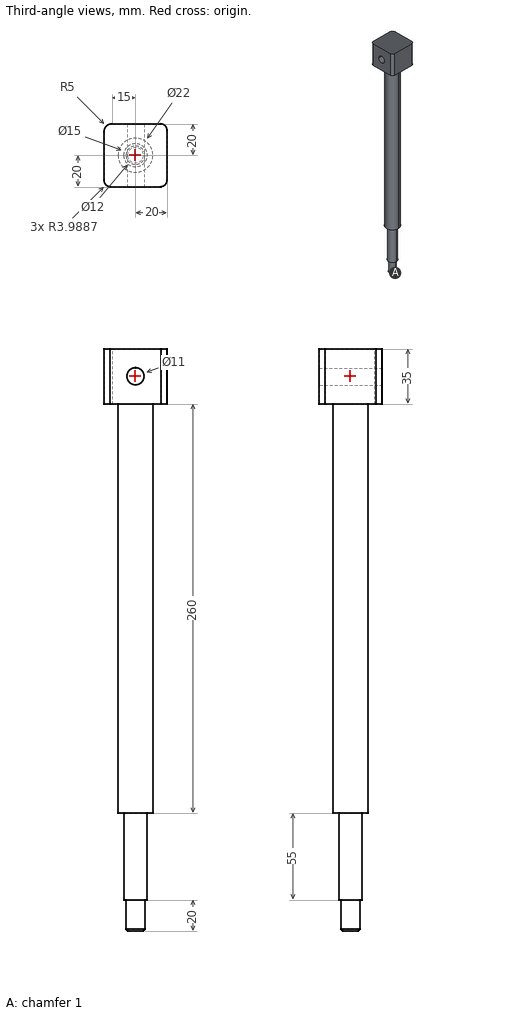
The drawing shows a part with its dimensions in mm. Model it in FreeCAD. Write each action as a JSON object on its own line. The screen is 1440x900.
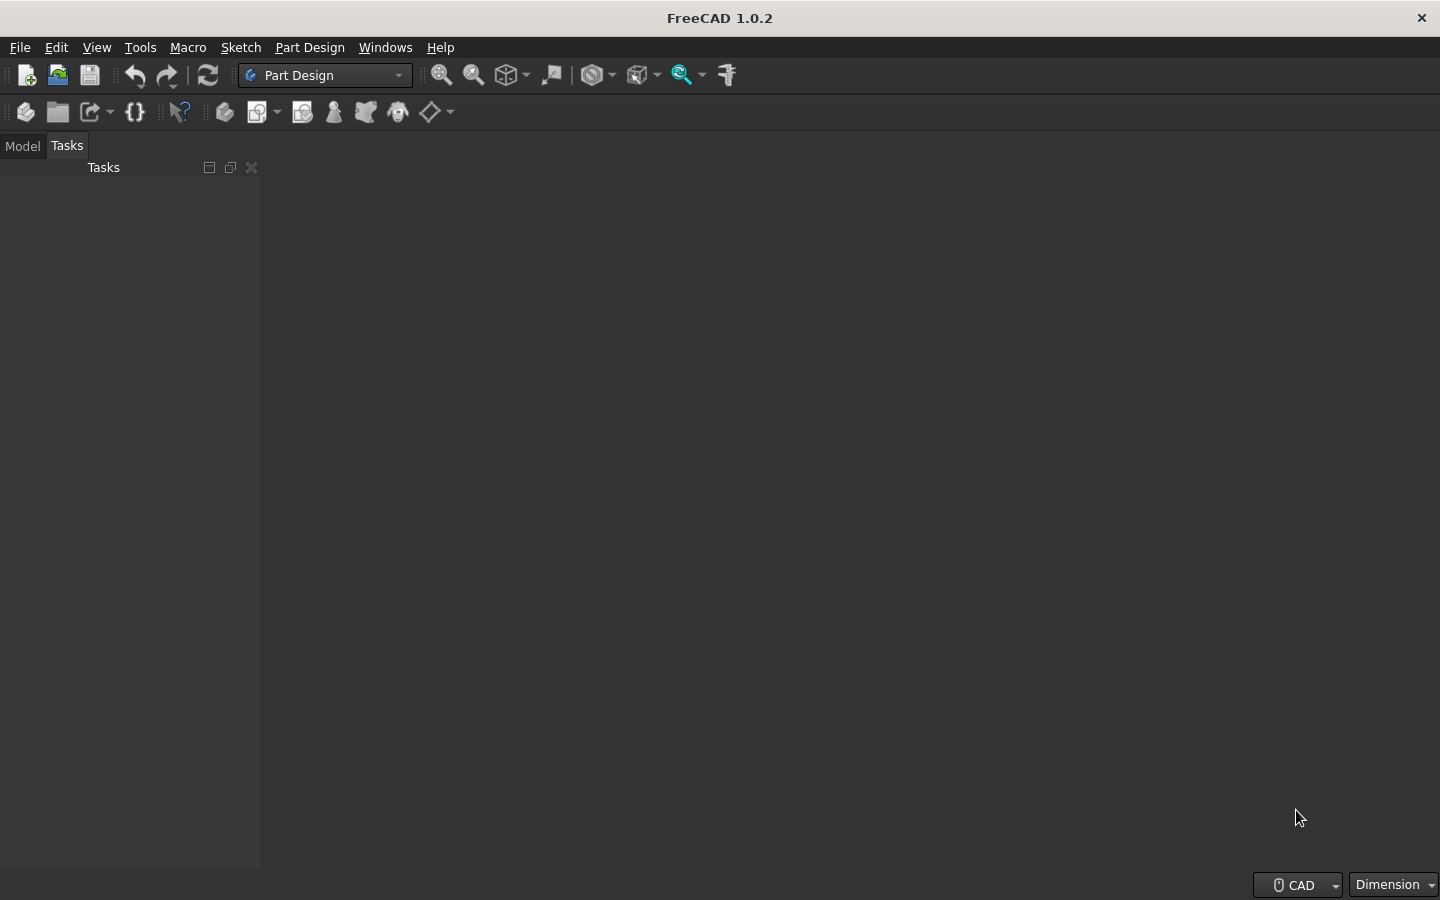
{"action": "left_click", "coordinate": [26, 76]}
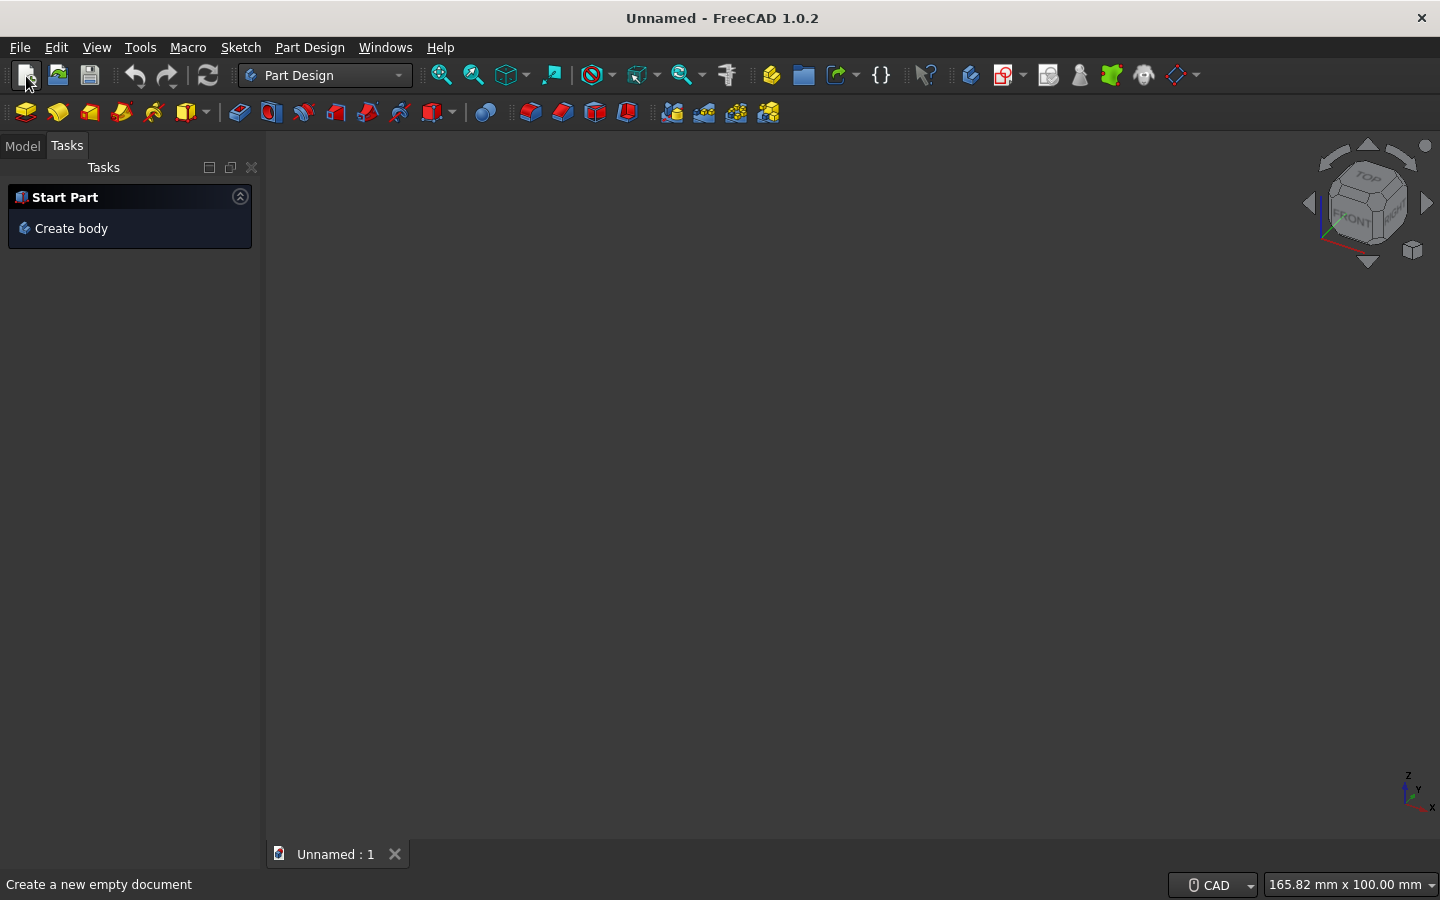
{"action": "left_click", "coordinate": [1004, 76]}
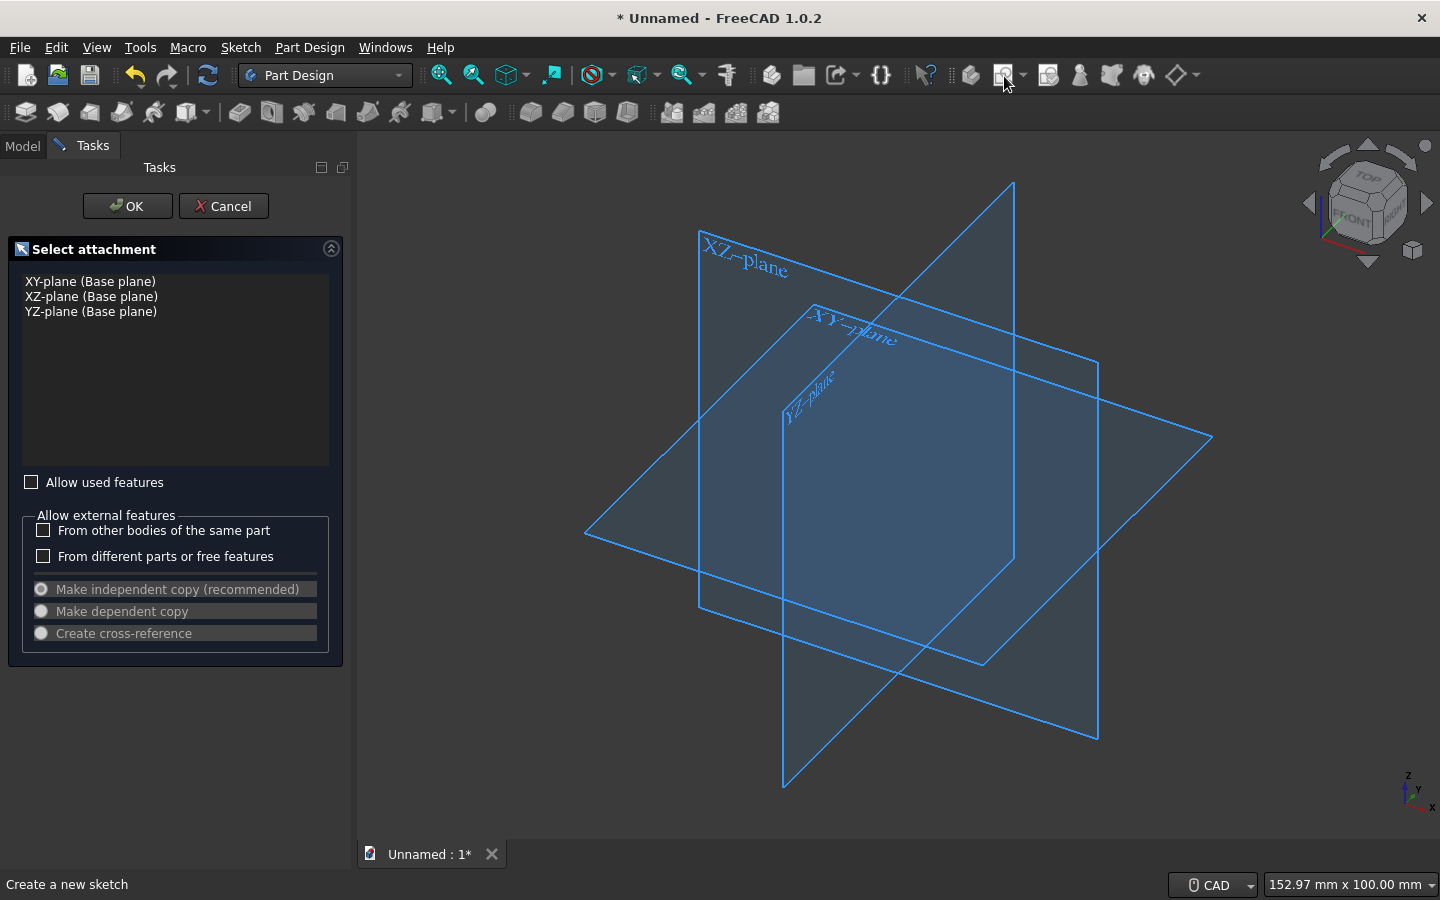
{"action": "left_click", "coordinate": [82, 282]}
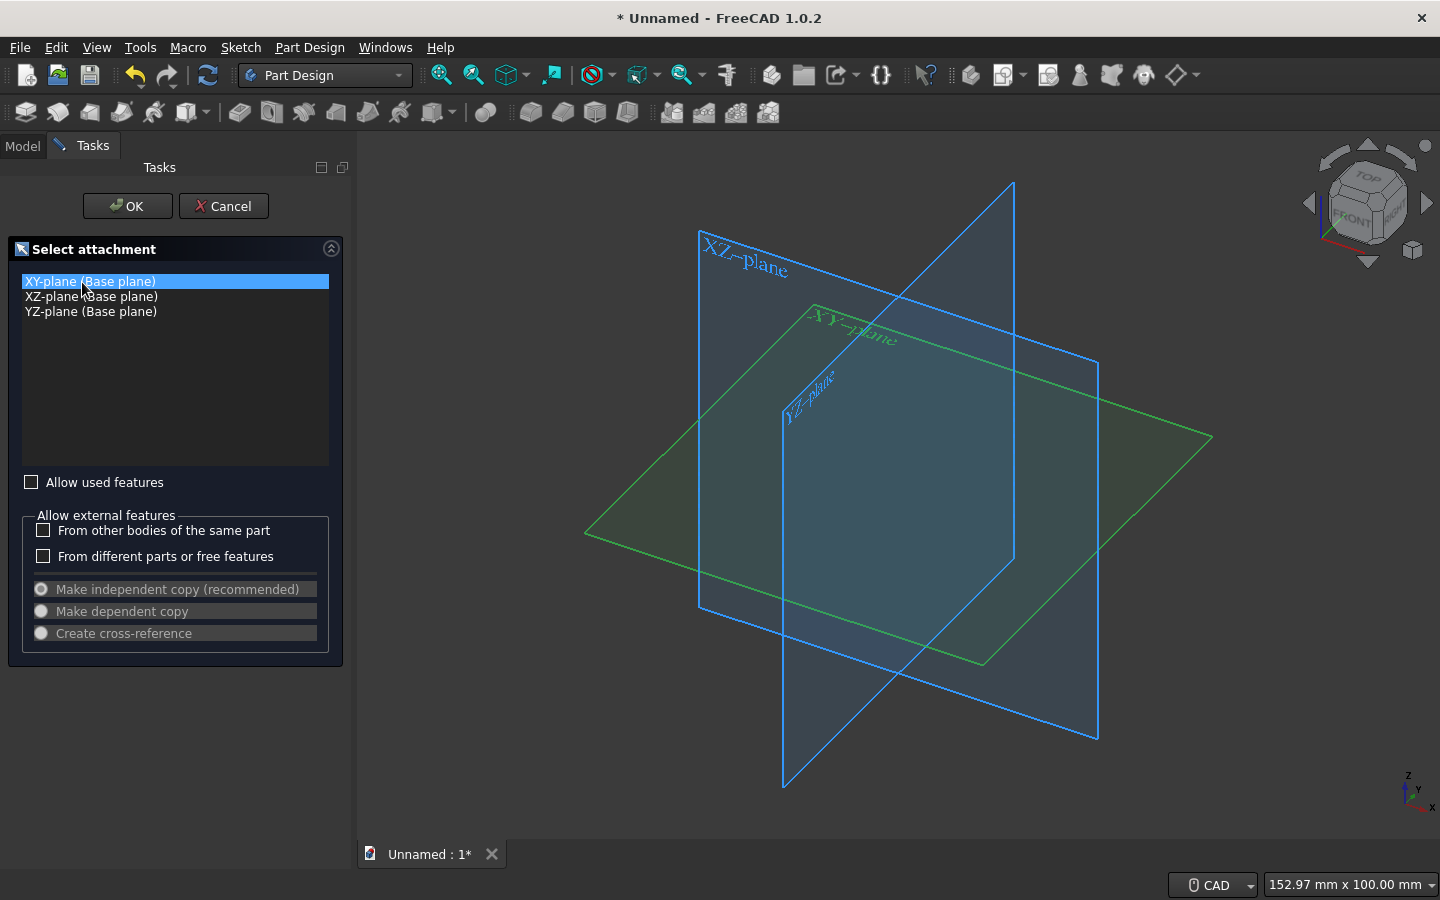
{"action": "left_click", "coordinate": [128, 206]}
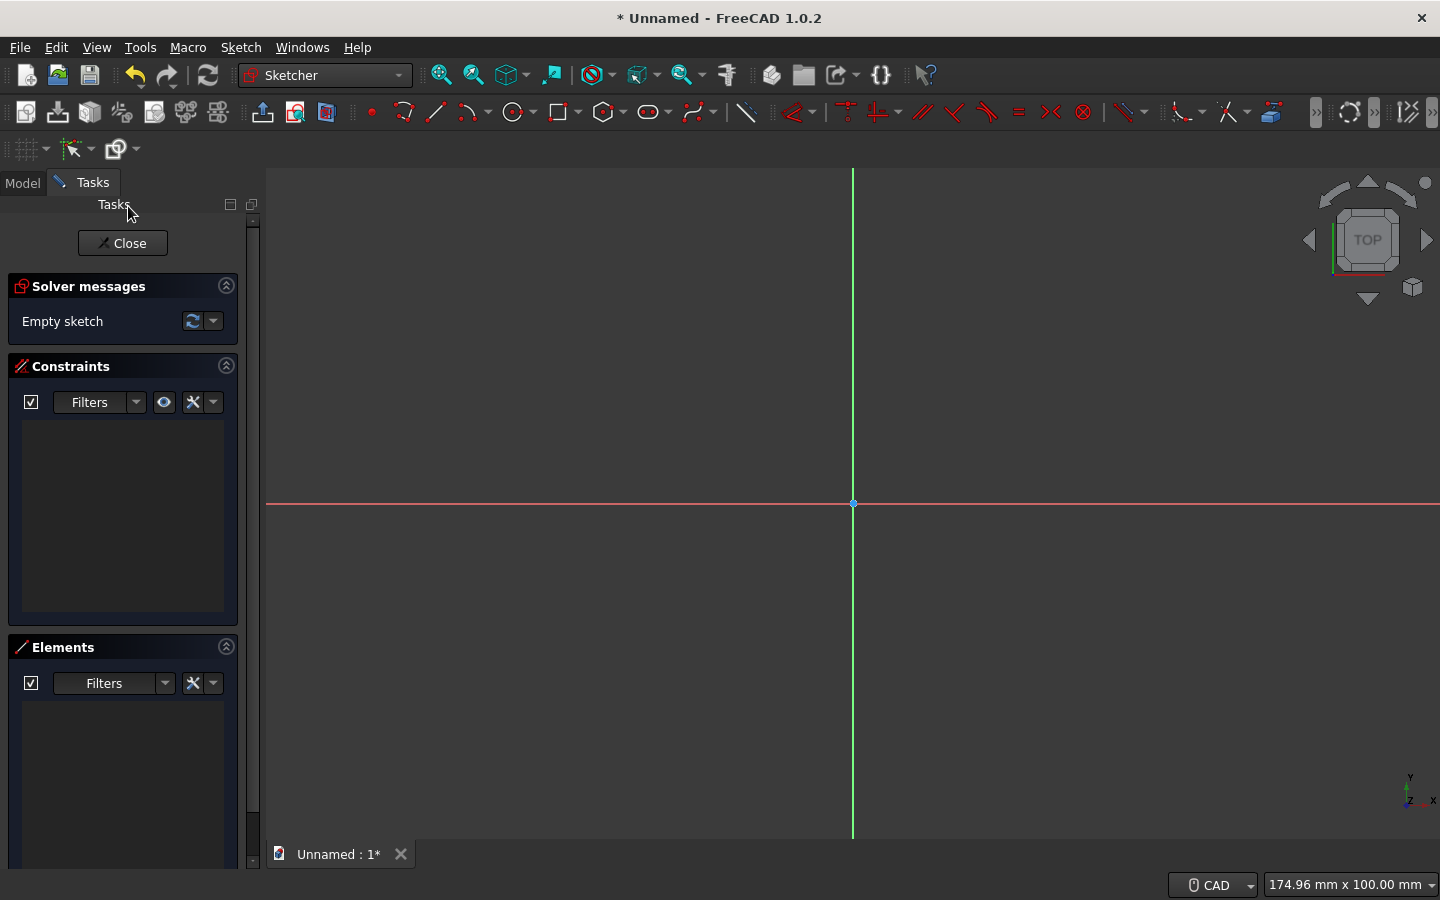
{"action": "scroll", "coordinate": [992, 504], "scroll_direction": "up", "scroll_amount": 2}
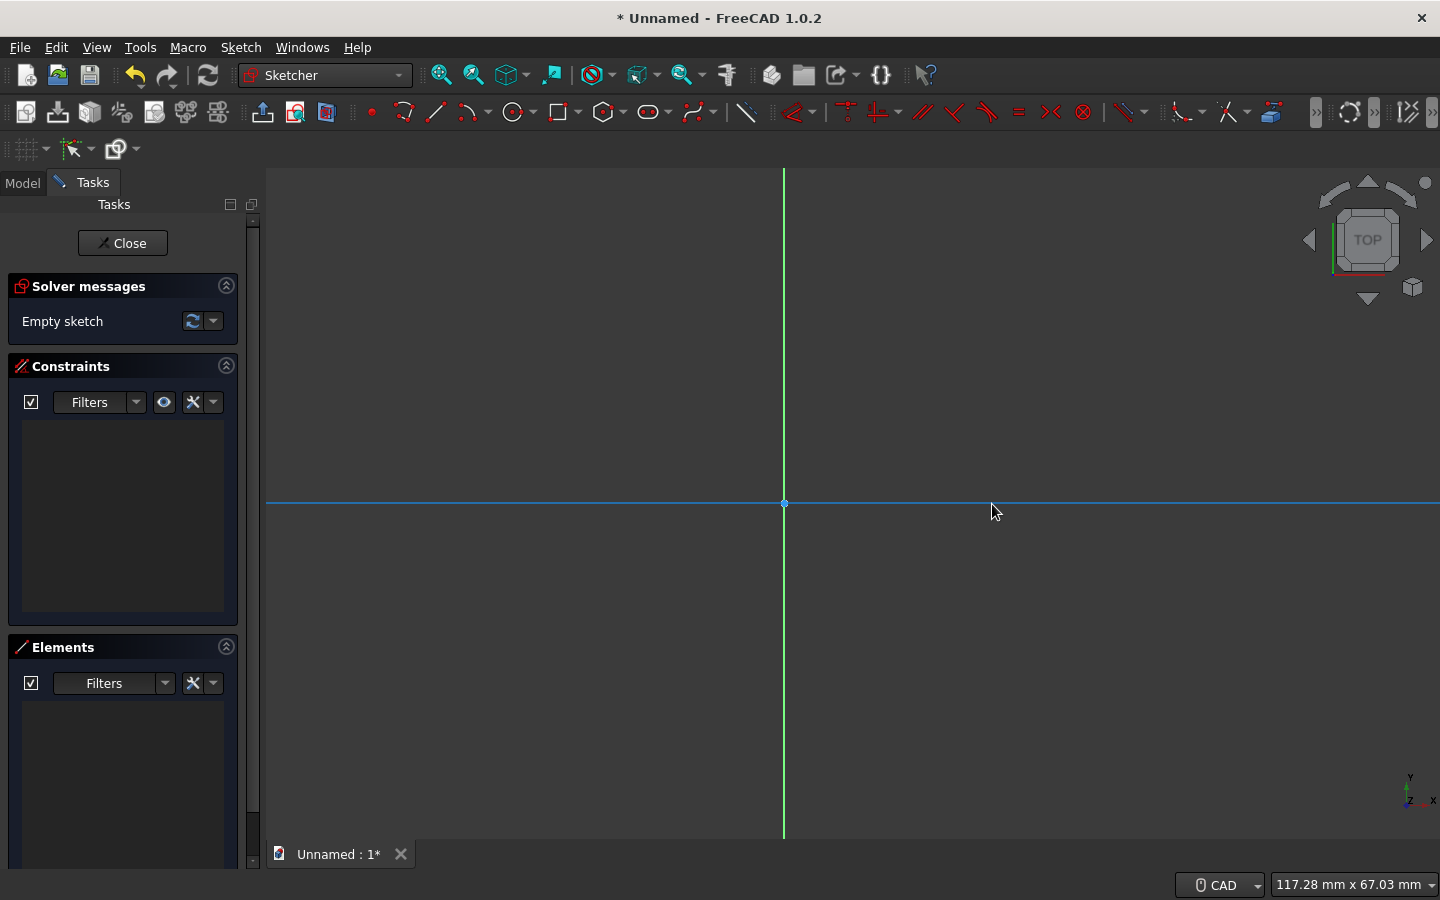
{"action": "key", "text": "g l"}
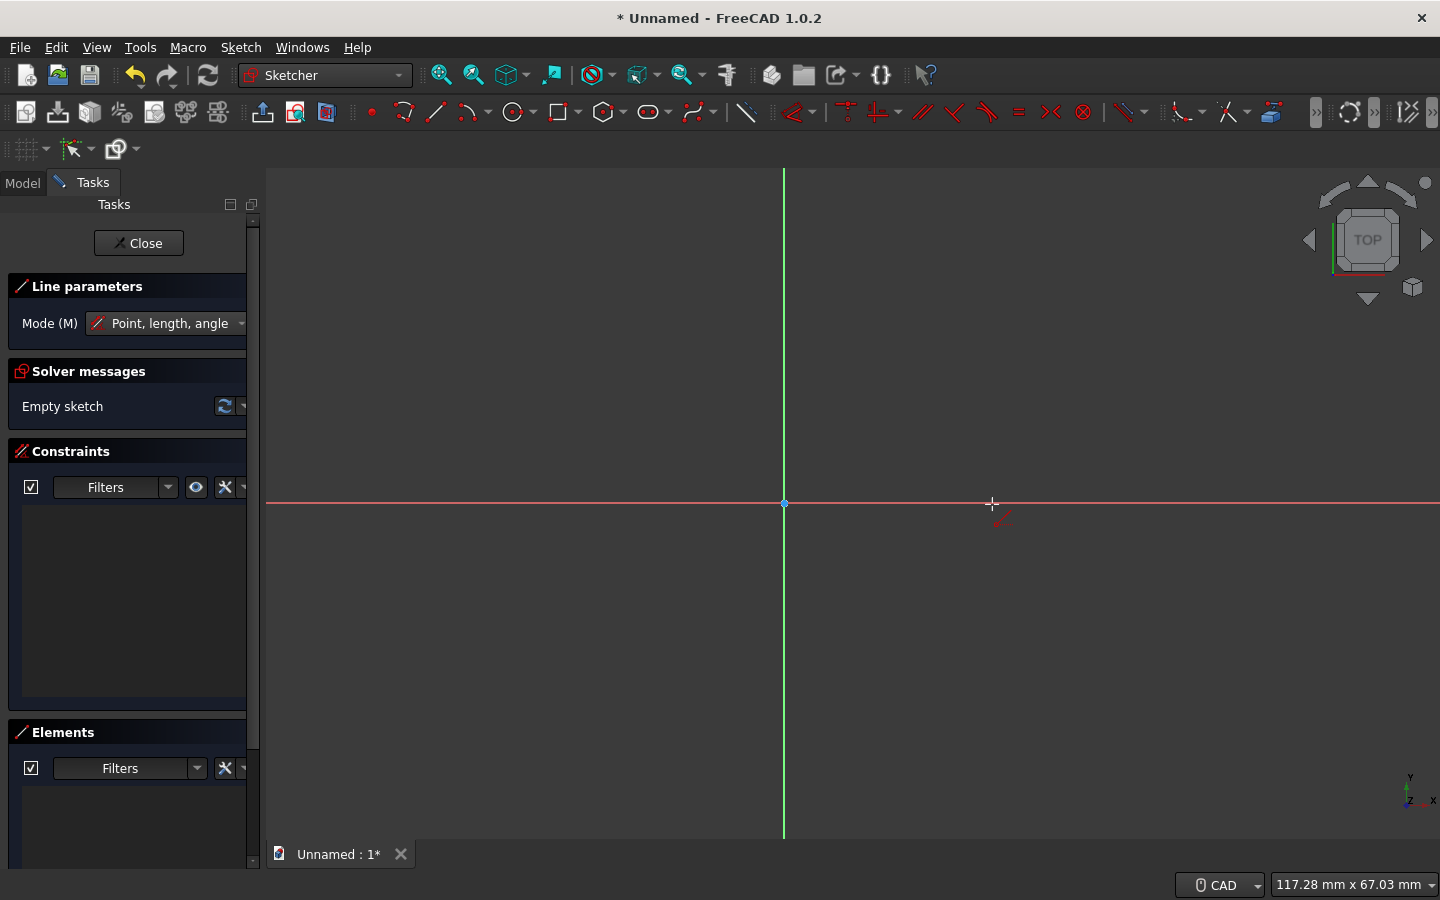
{"action": "left_click", "coordinate": [945, 303]}
{"action": "left_click", "coordinate": [634, 303]}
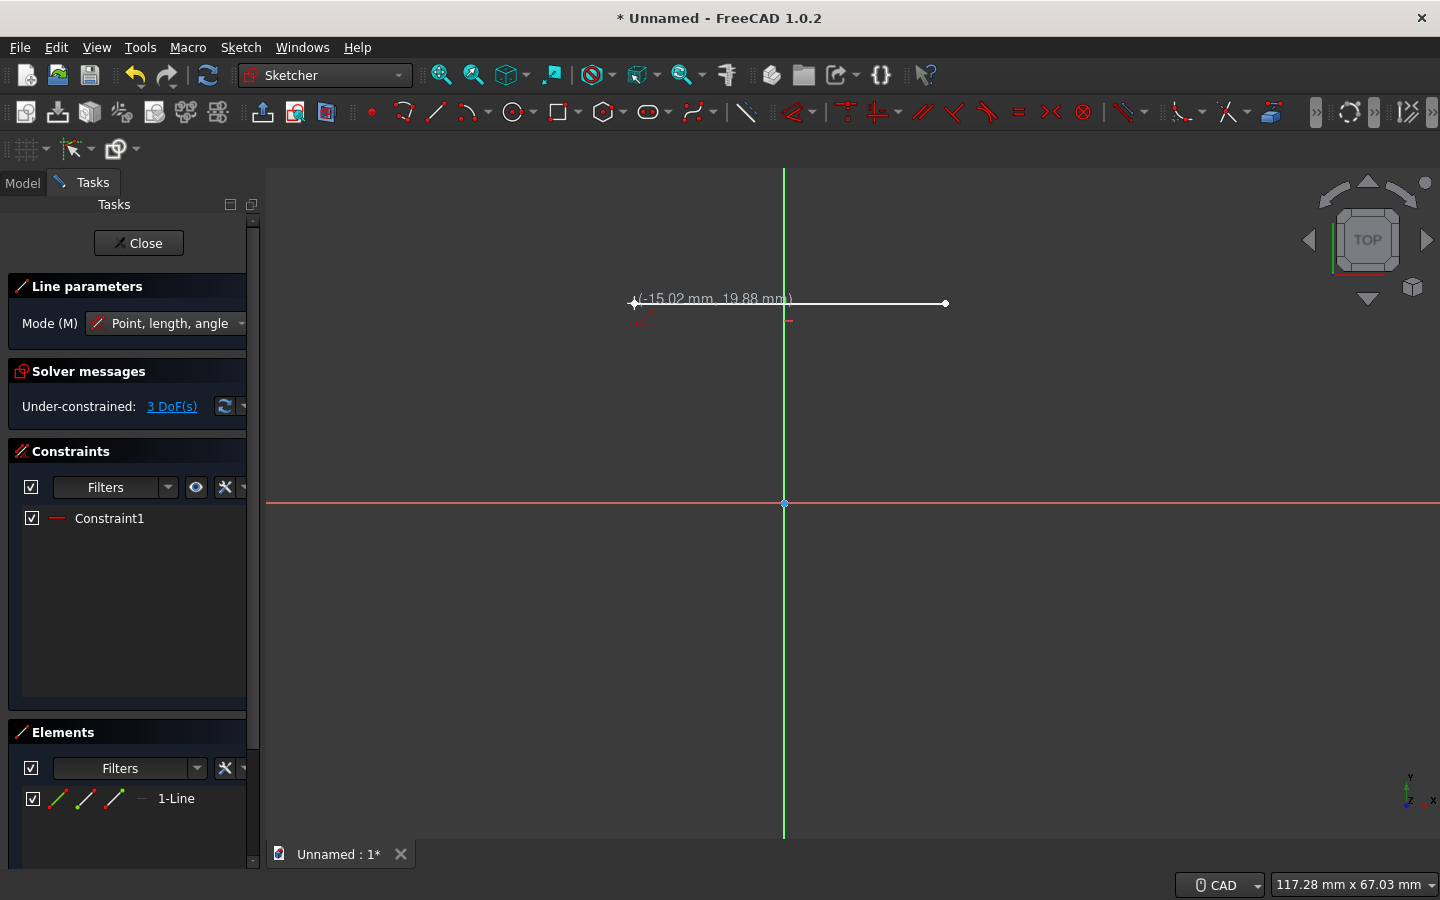
{"action": "left_click", "coordinate": [584, 353]}
{"action": "left_click", "coordinate": [584, 663]}